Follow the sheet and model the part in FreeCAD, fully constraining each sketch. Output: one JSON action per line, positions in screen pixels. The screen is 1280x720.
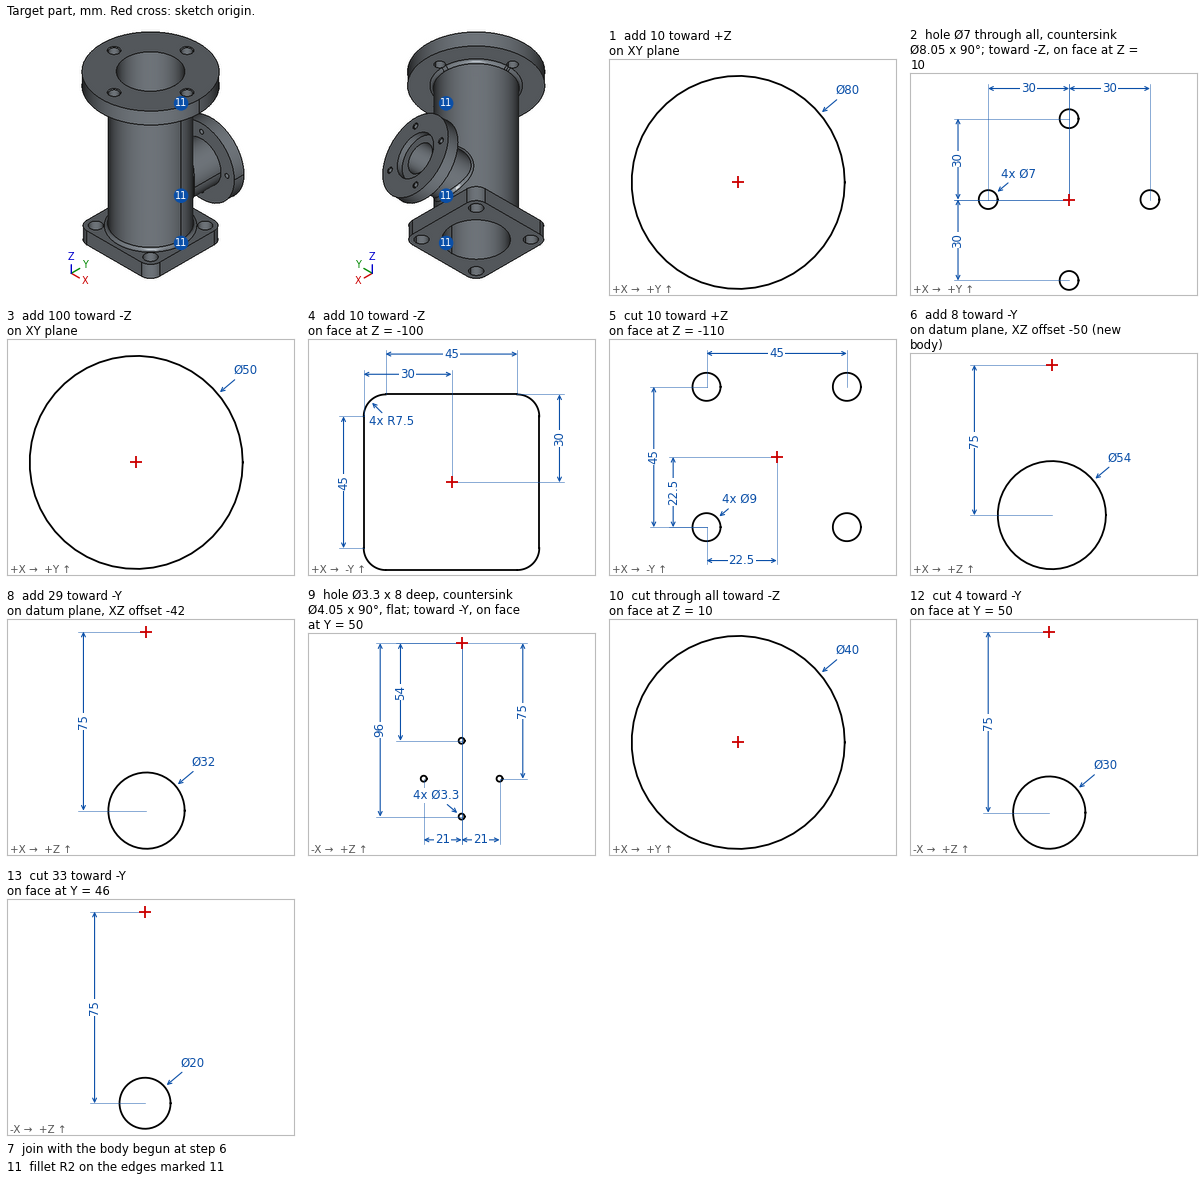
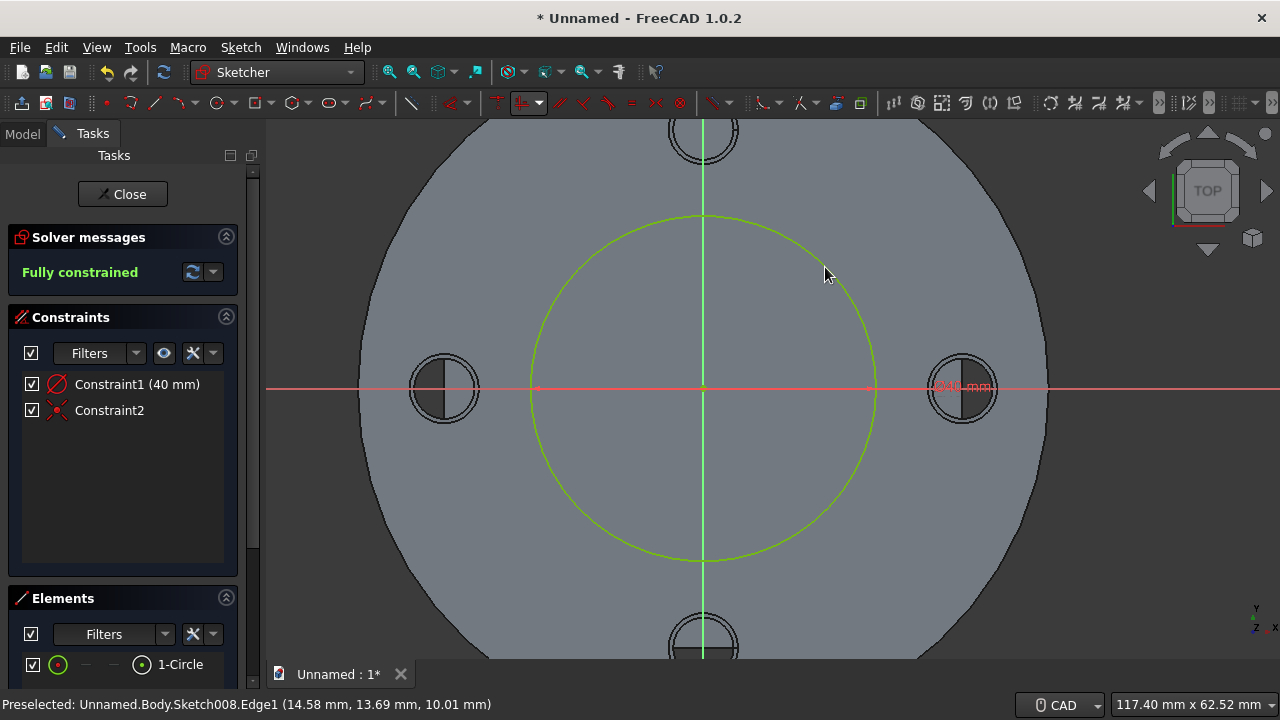
{"action": "left_click", "coordinate": [123, 194]}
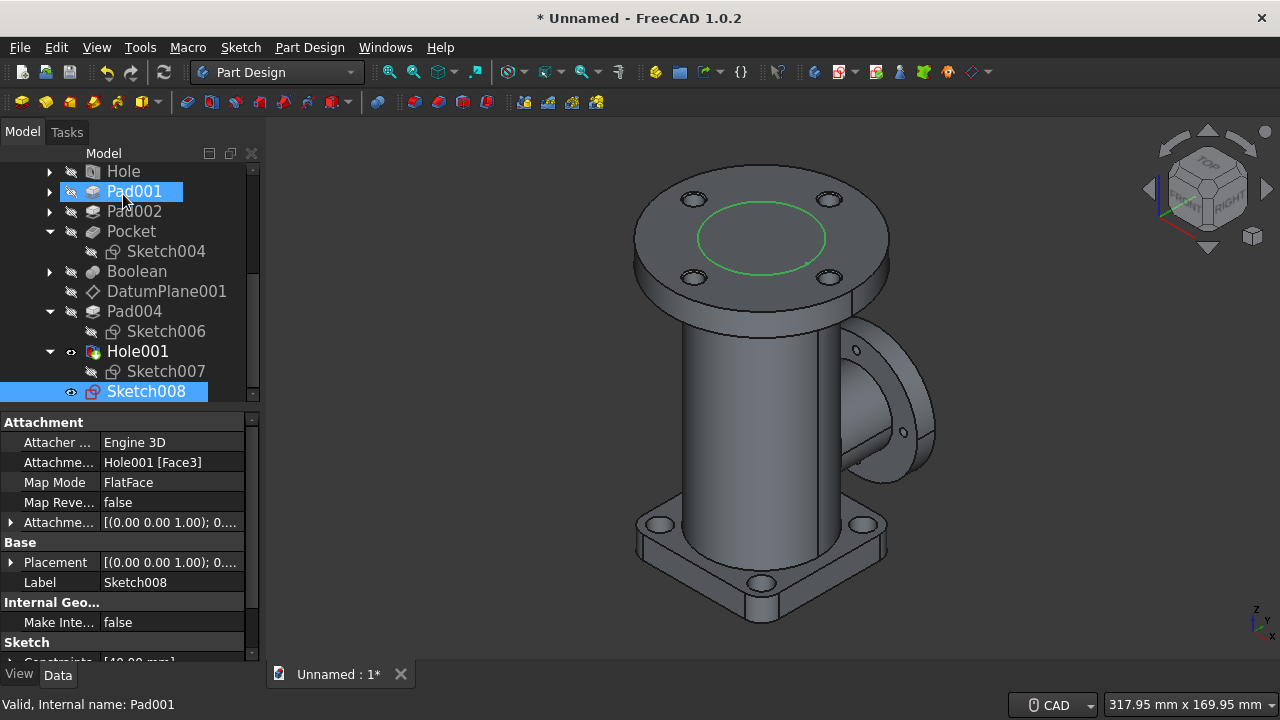
{"action": "left_click", "coordinate": [188, 102]}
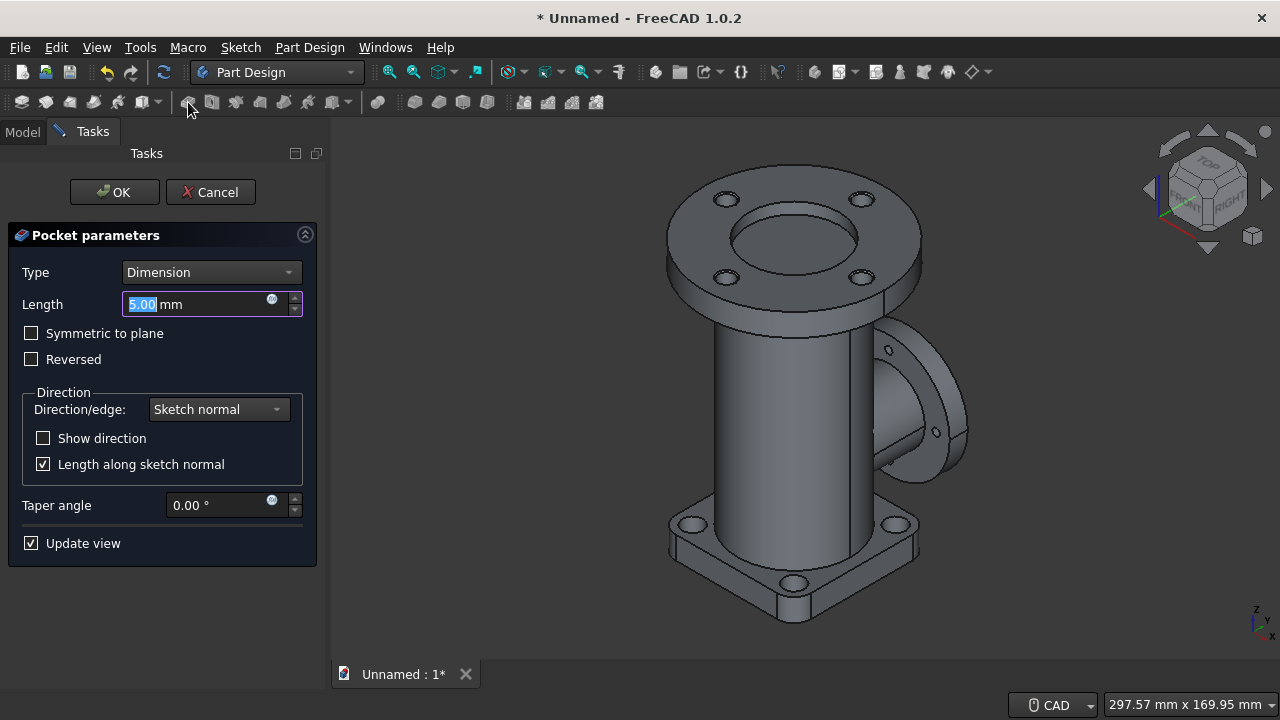
{"action": "left_click", "coordinate": [212, 272]}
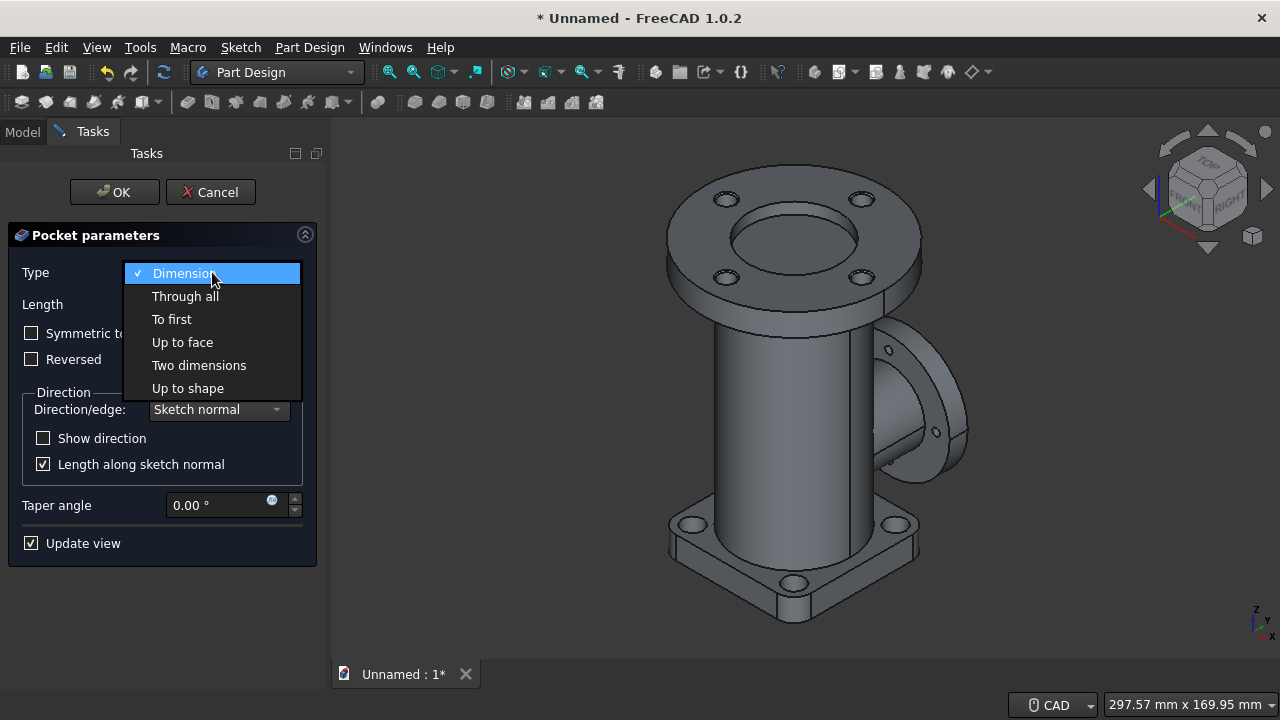
{"action": "left_click", "coordinate": [212, 296]}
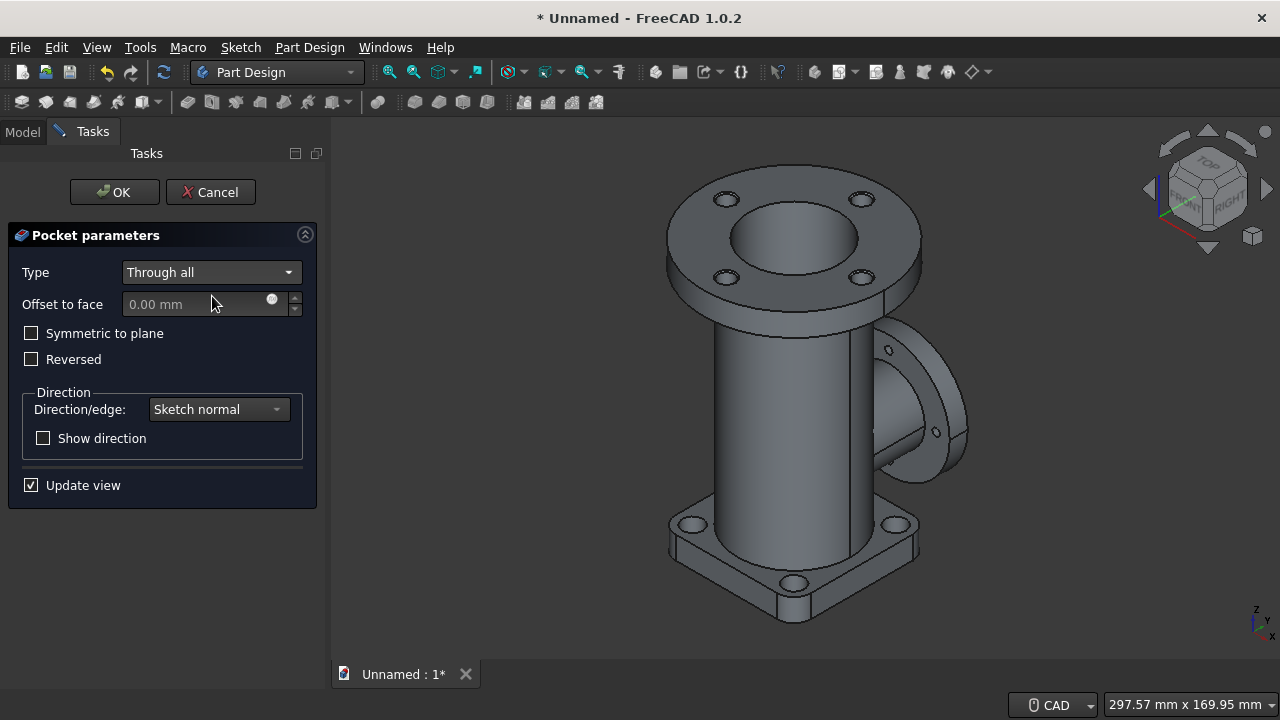
{"action": "left_click", "coordinate": [115, 192]}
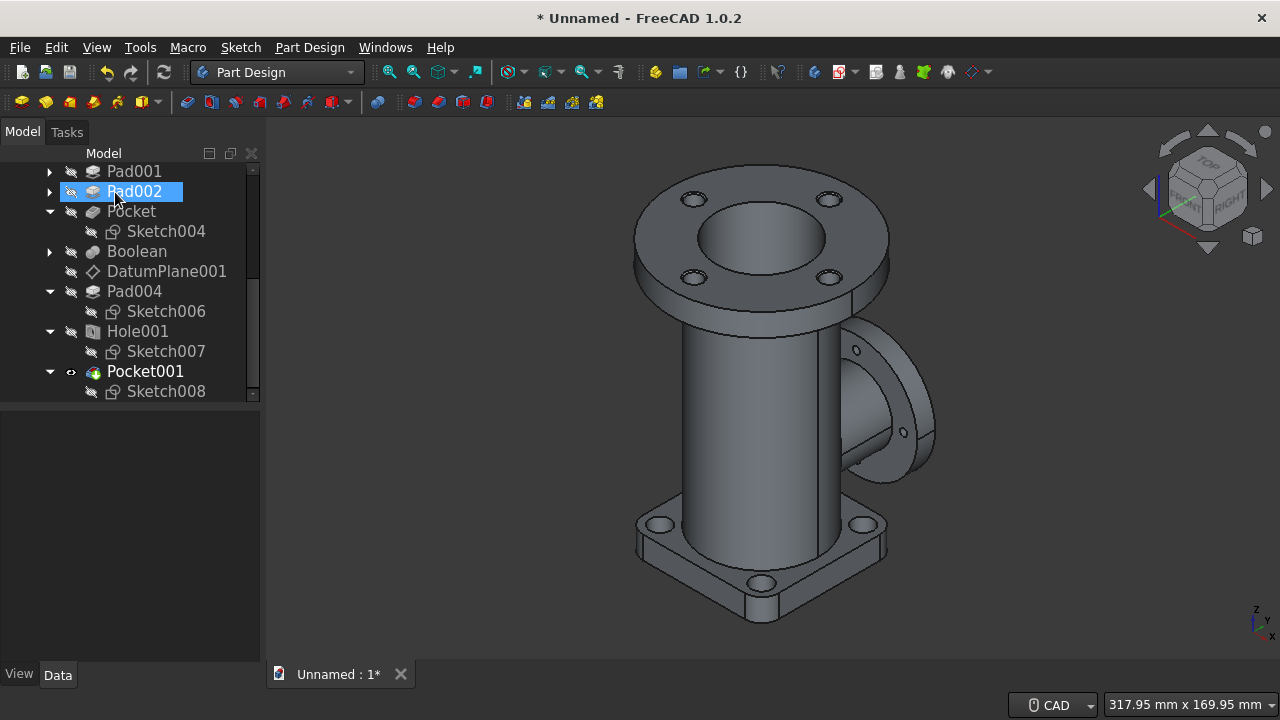
{"action": "left_click", "coordinate": [719, 395]}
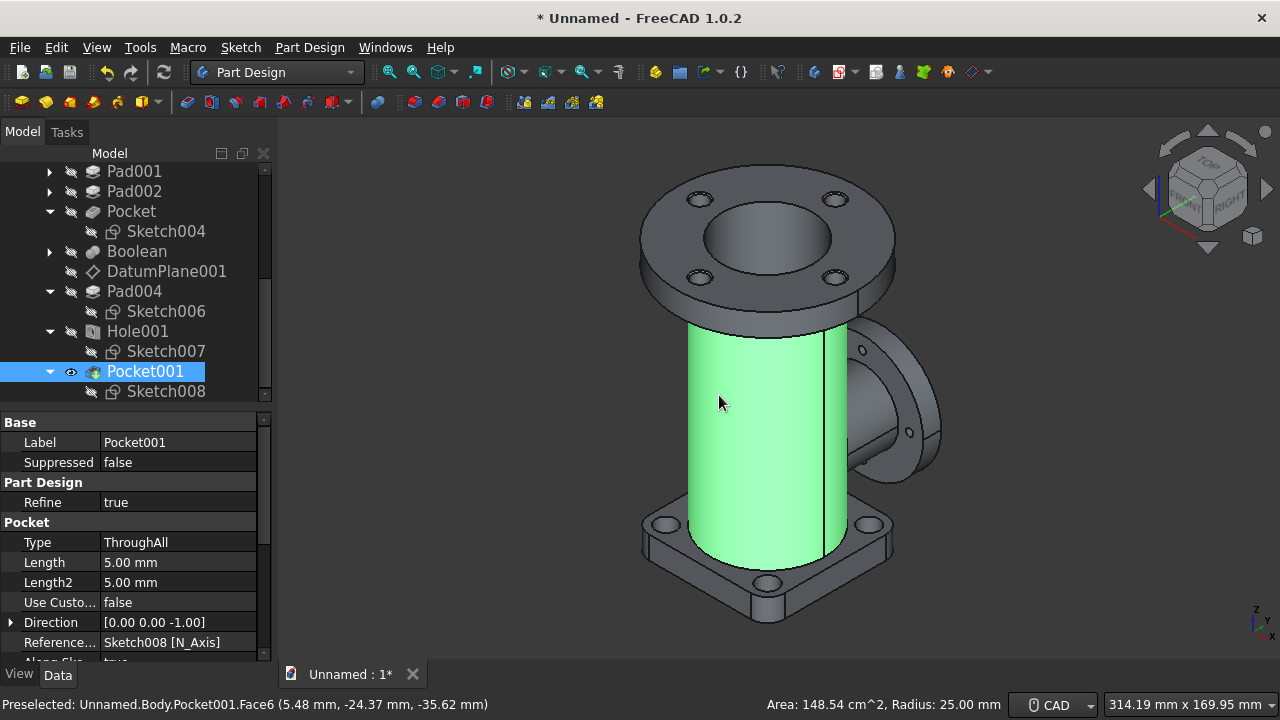
{"action": "left_click", "coordinate": [416, 102]}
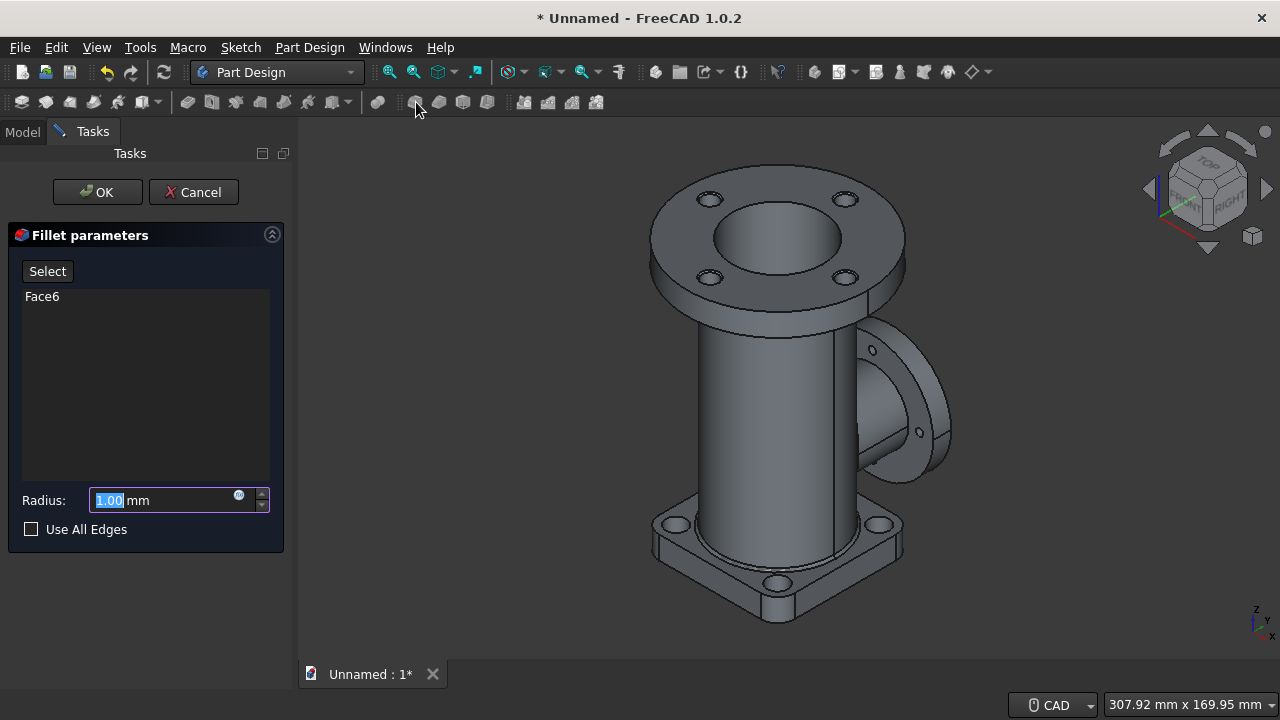
{"action": "type", "text": "2"}
{"action": "key", "text": "Tab"}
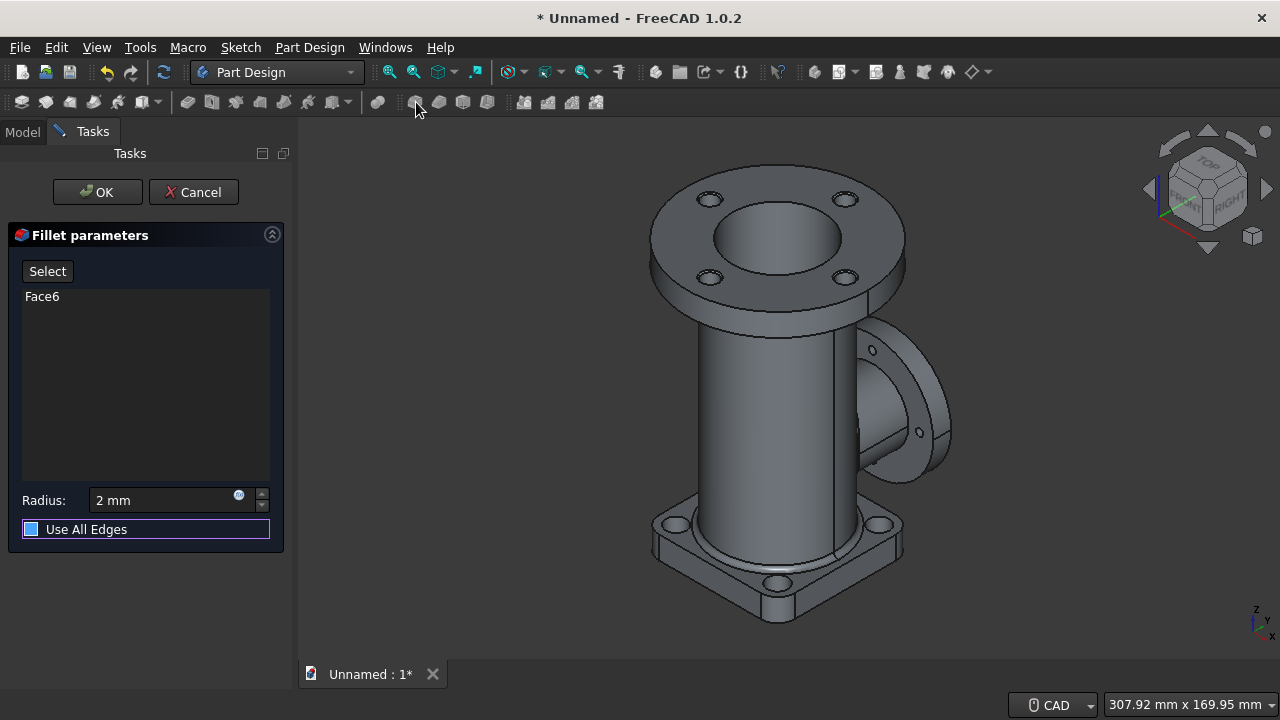
{"action": "left_click", "coordinate": [98, 192]}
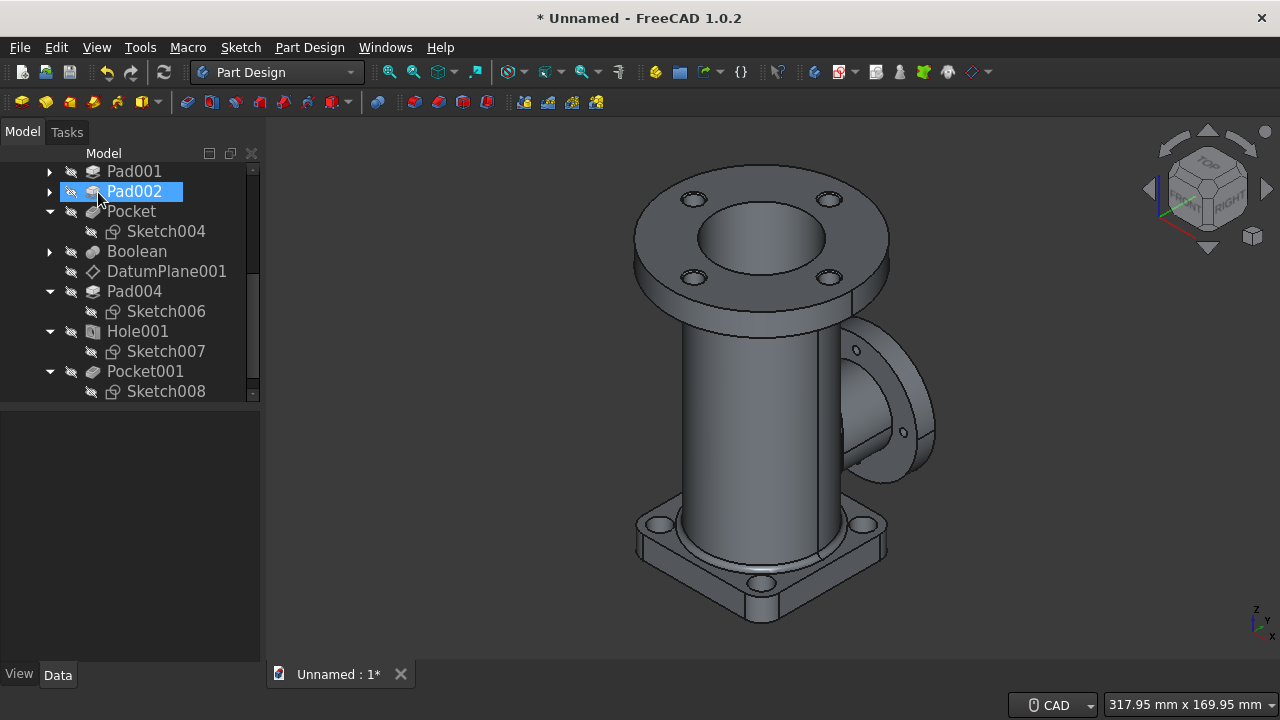
{"action": "key", "text": "4"}